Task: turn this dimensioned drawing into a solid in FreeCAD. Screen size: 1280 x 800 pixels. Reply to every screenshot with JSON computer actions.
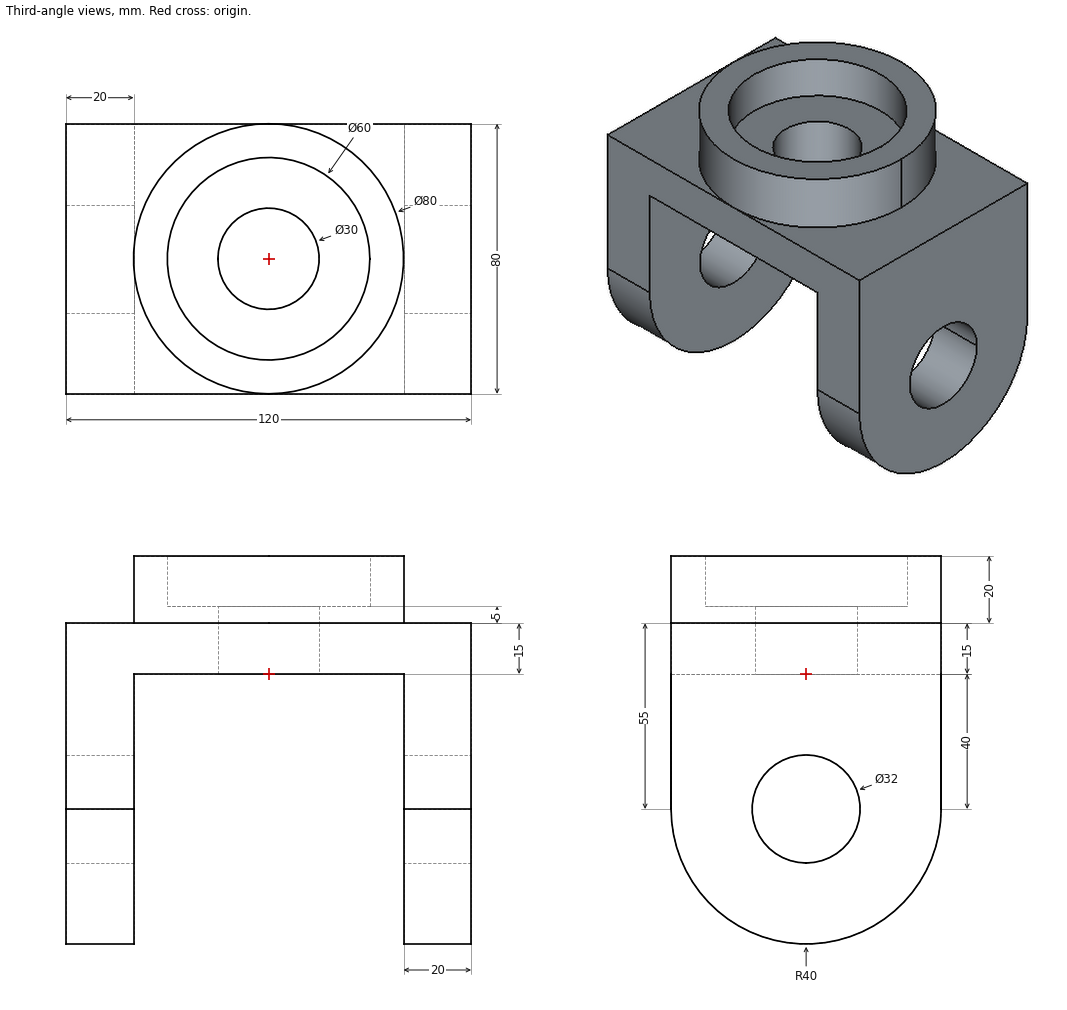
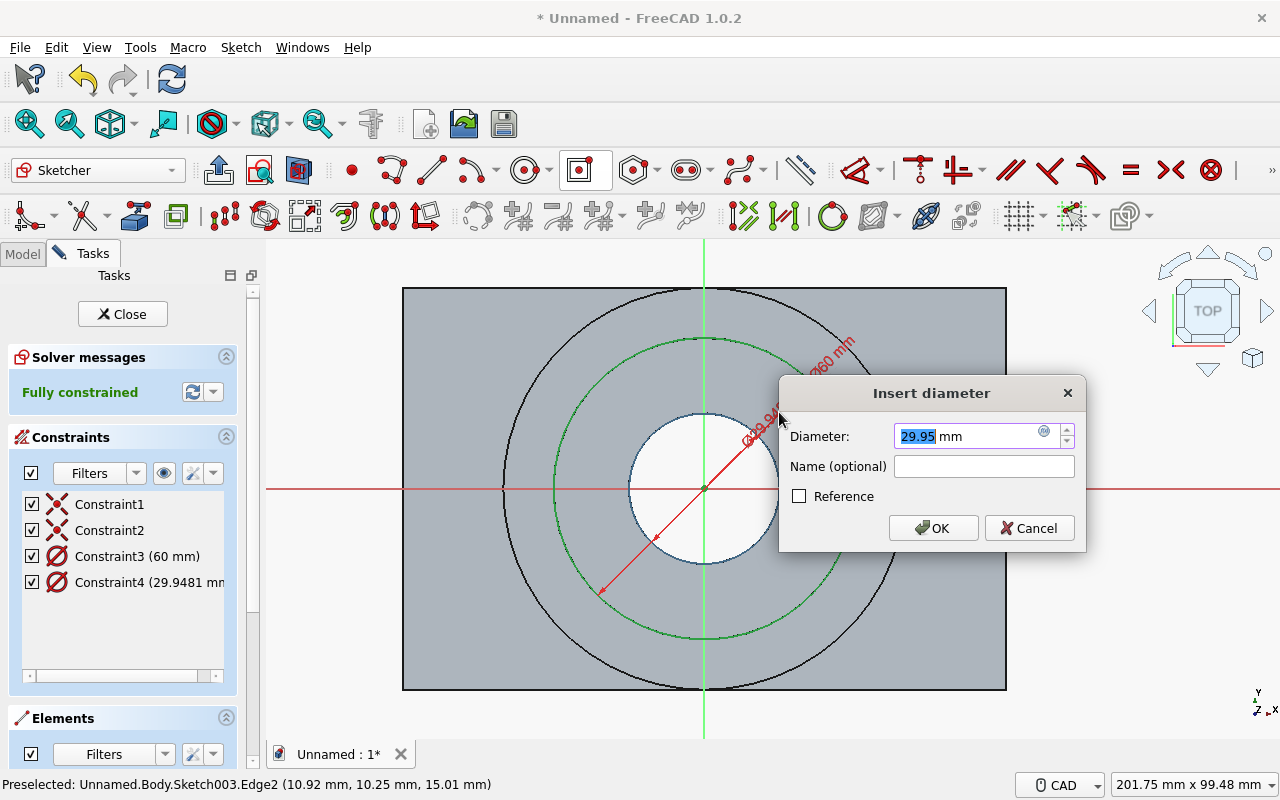
{"action": "type", "text": "30"}
{"action": "key", "text": "Return"}
{"action": "key", "text": "Escape"}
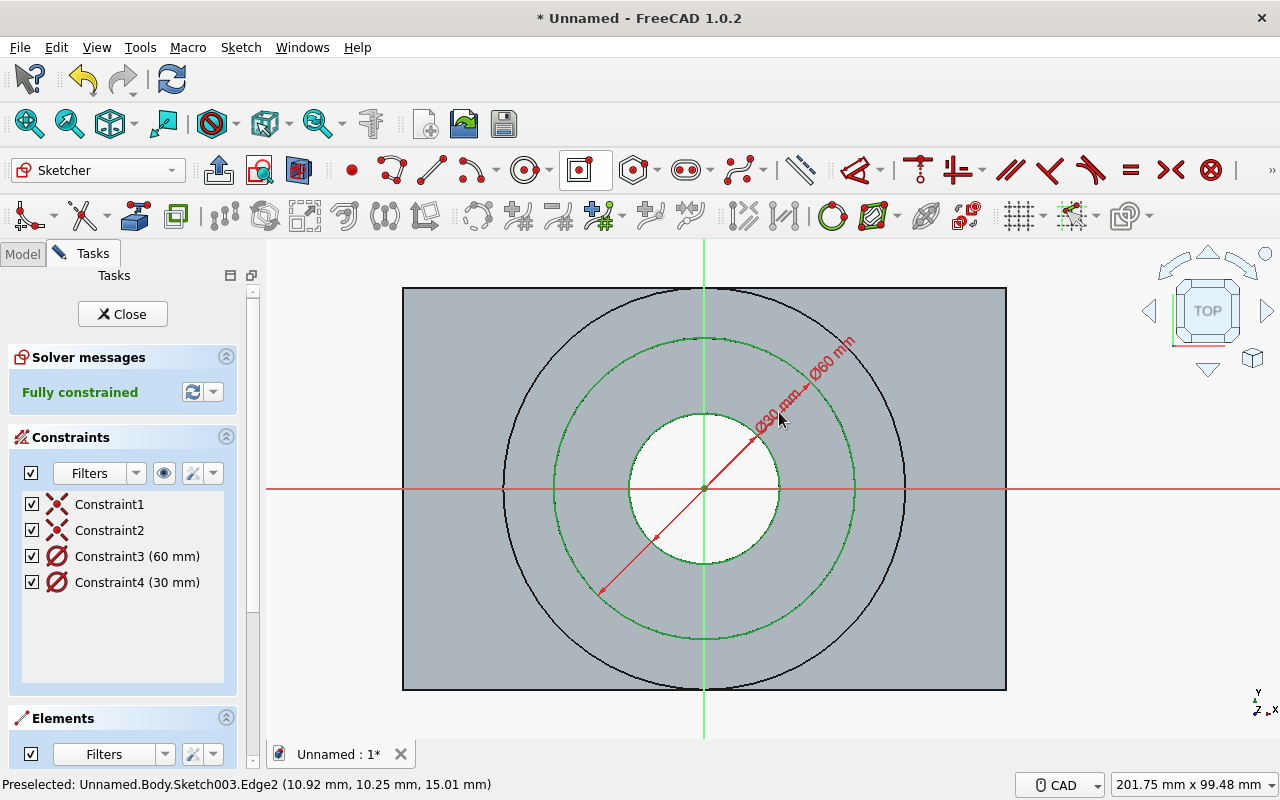
{"action": "left_click", "coordinate": [123, 314]}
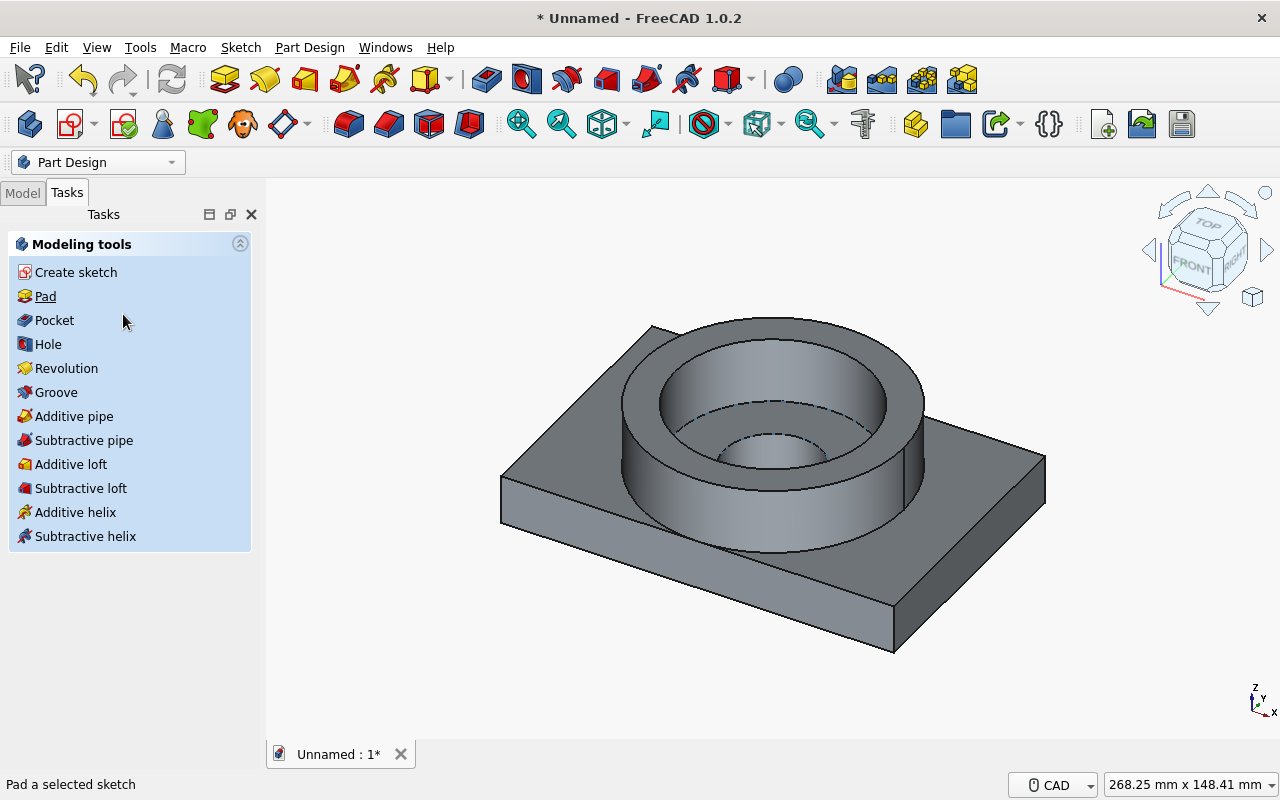
{"action": "left_click", "coordinate": [226, 80]}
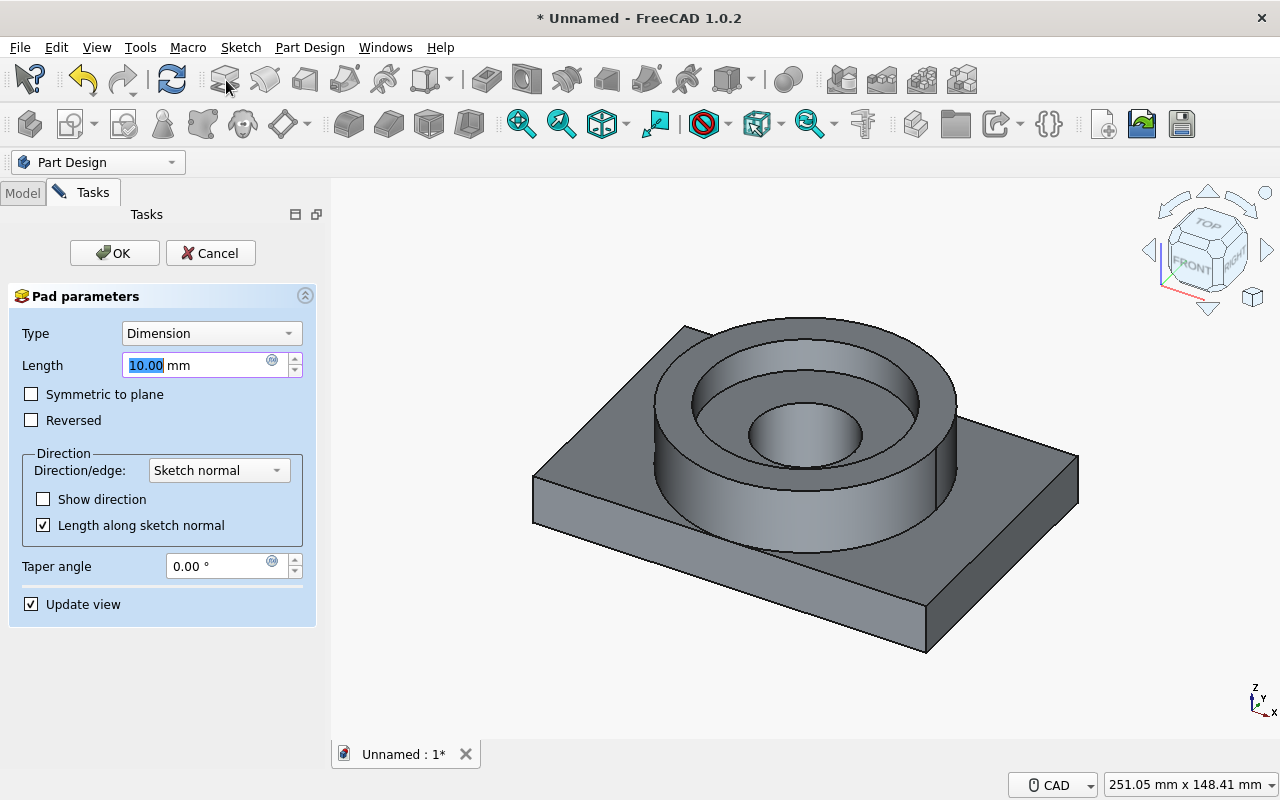
{"action": "type", "text": "5"}
{"action": "key", "text": "Tab"}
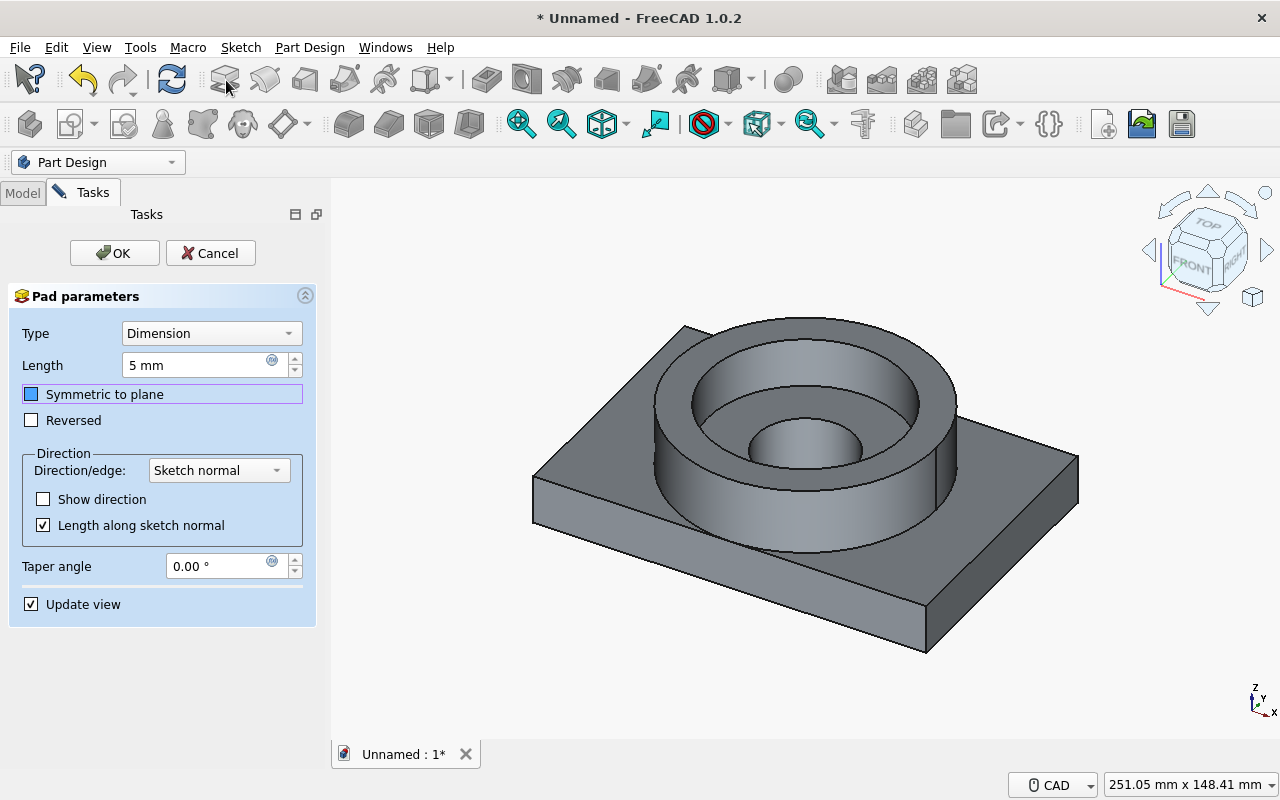
{"action": "left_click", "coordinate": [115, 253]}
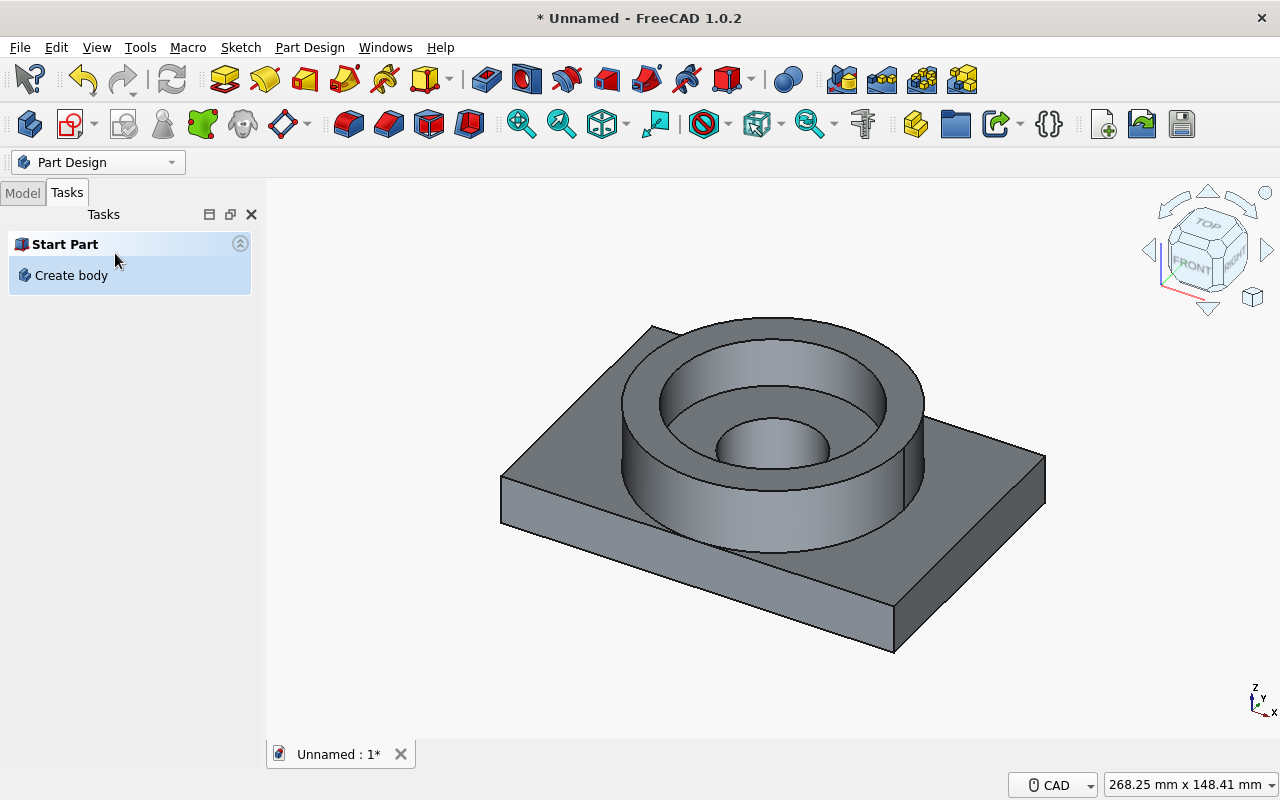
{"action": "left_click", "coordinate": [1013, 511]}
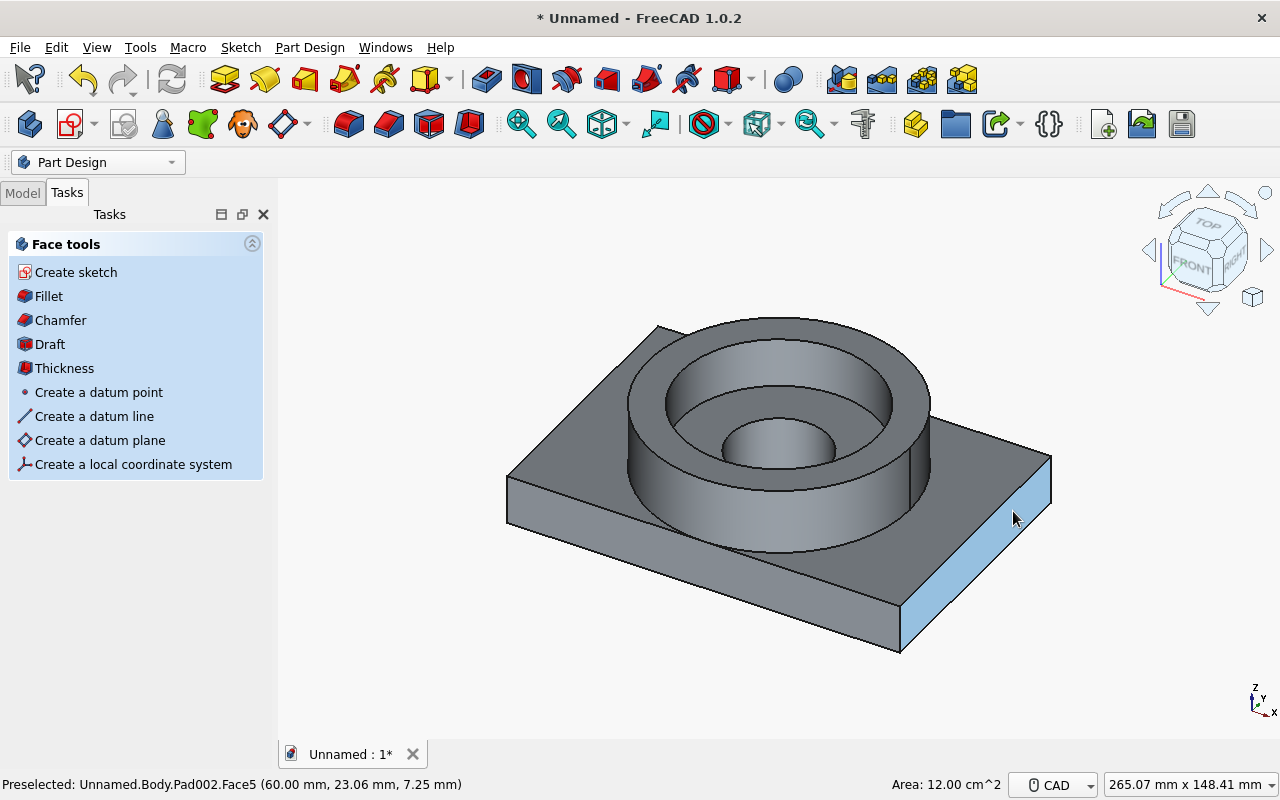
{"action": "left_click", "coordinate": [70, 124]}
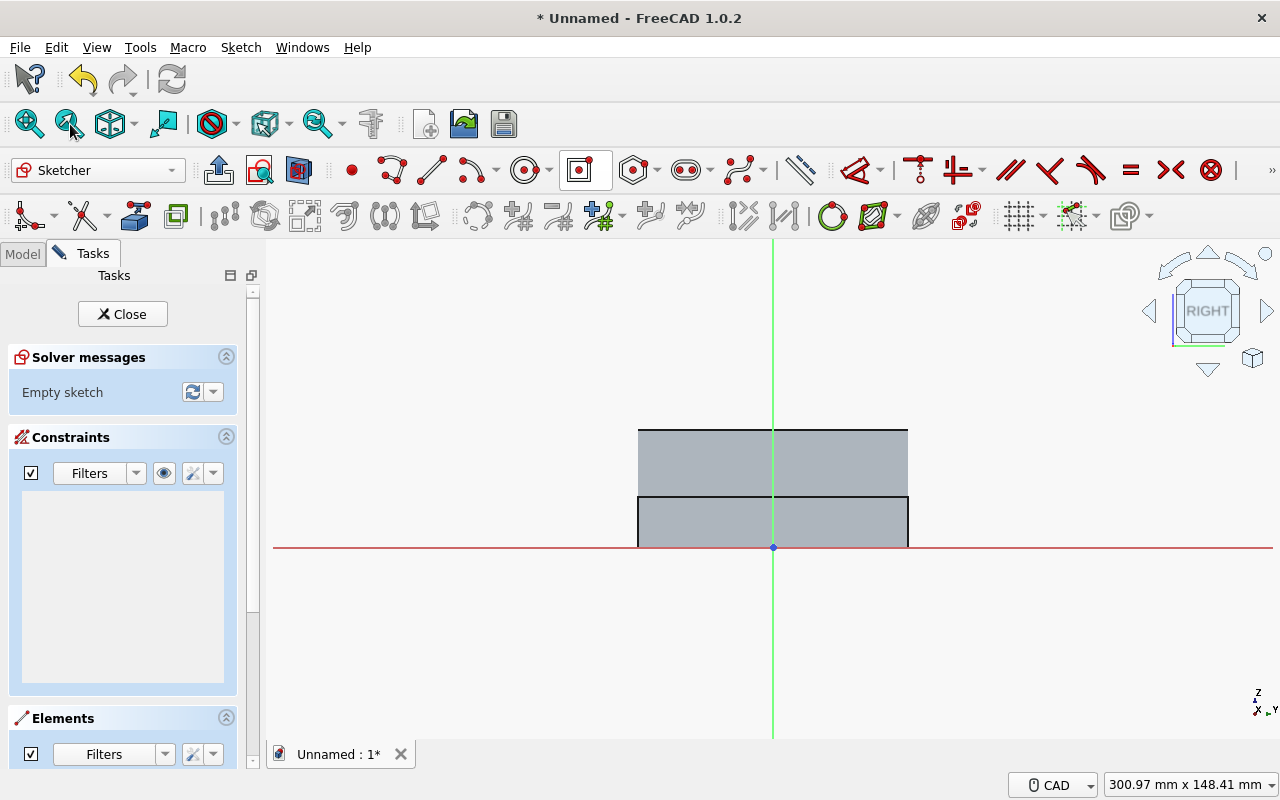
{"action": "scroll", "coordinate": [565, 267], "scroll_direction": "down", "scroll_amount": 2}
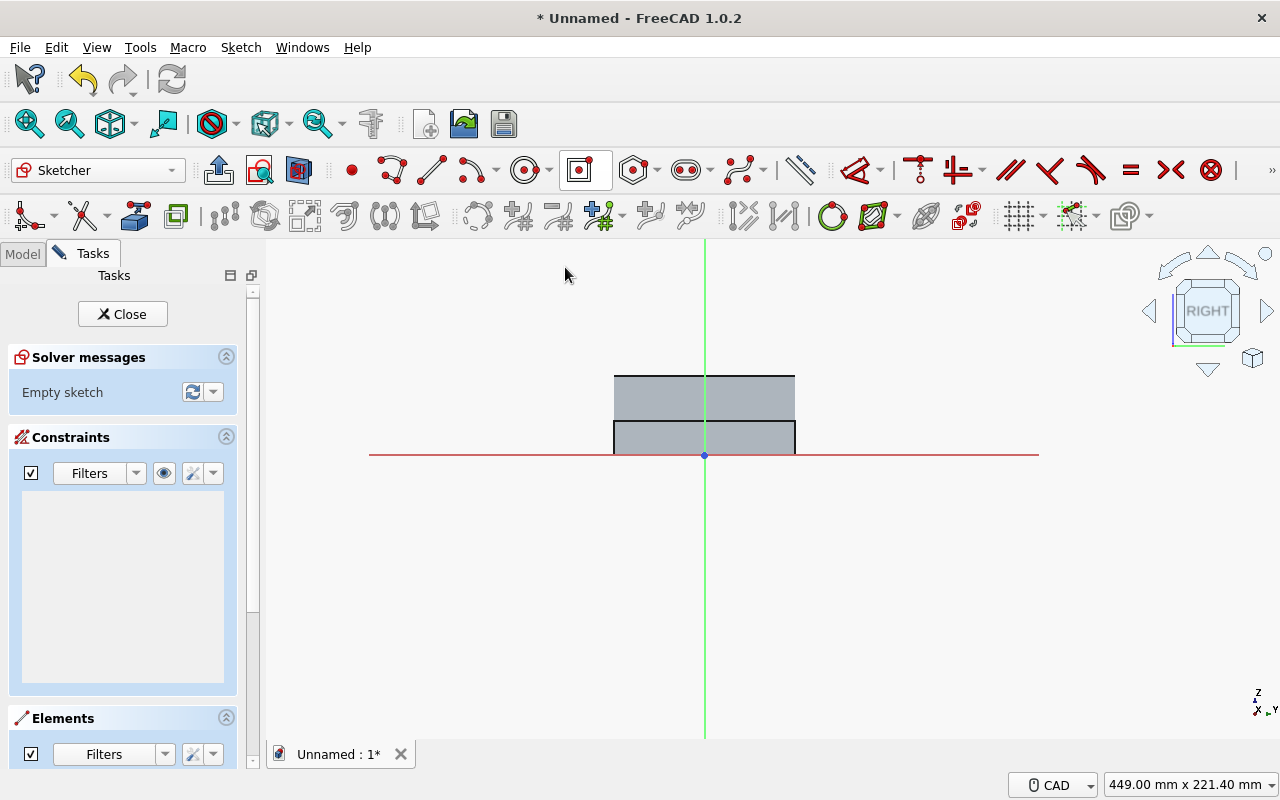
{"action": "scroll", "coordinate": [705, 615], "scroll_direction": "up", "scroll_amount": 3}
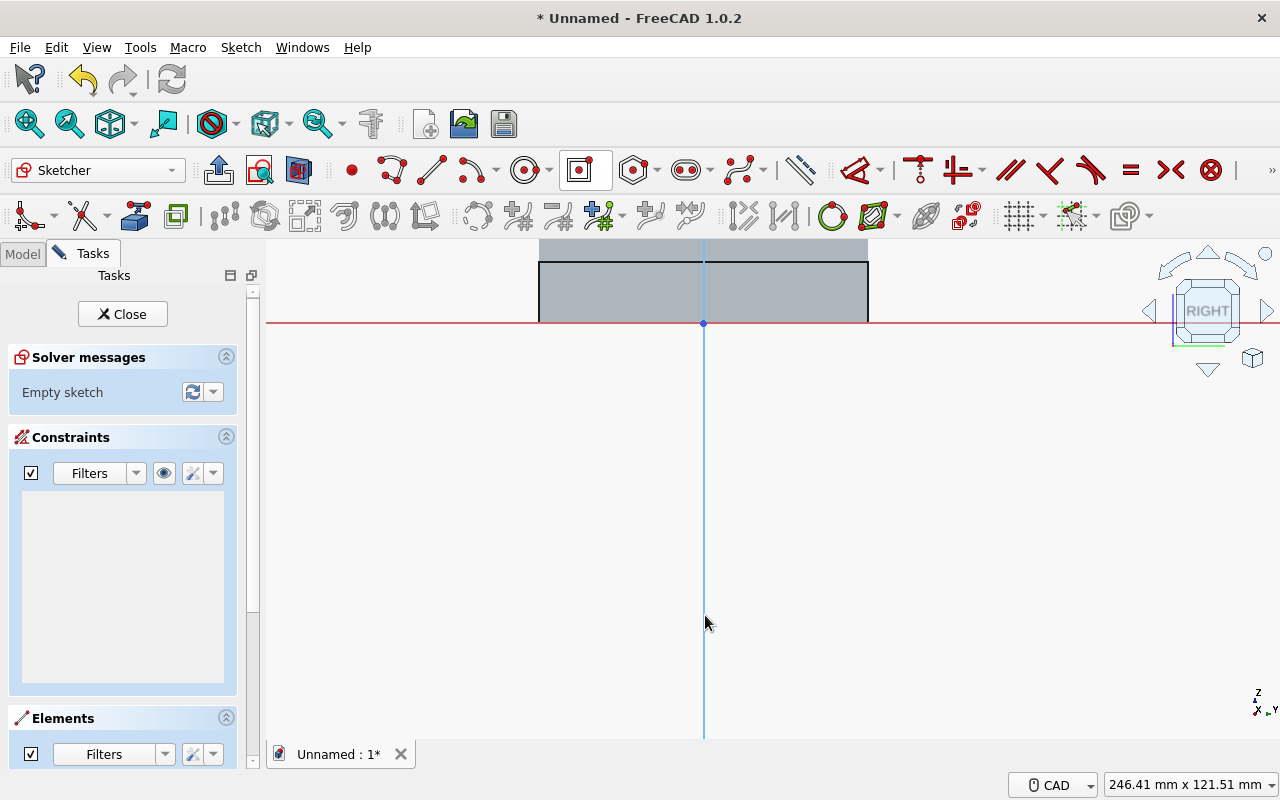
{"action": "left_click", "coordinate": [392, 170]}